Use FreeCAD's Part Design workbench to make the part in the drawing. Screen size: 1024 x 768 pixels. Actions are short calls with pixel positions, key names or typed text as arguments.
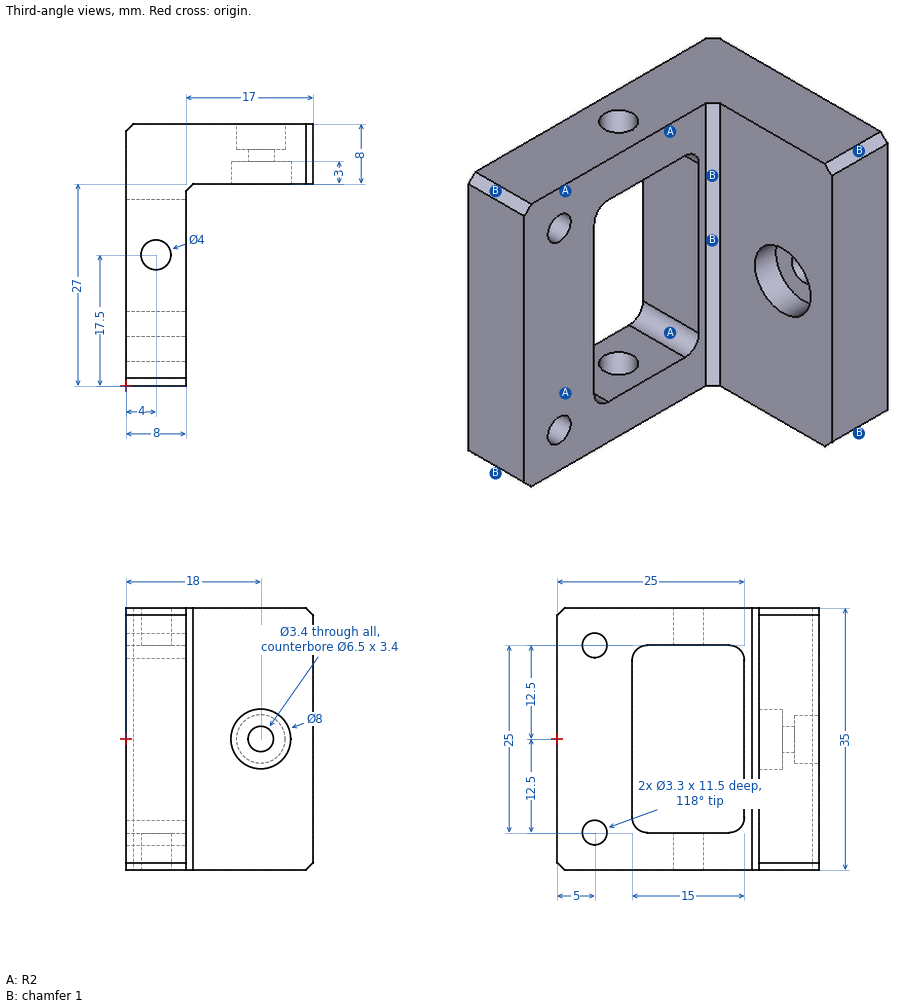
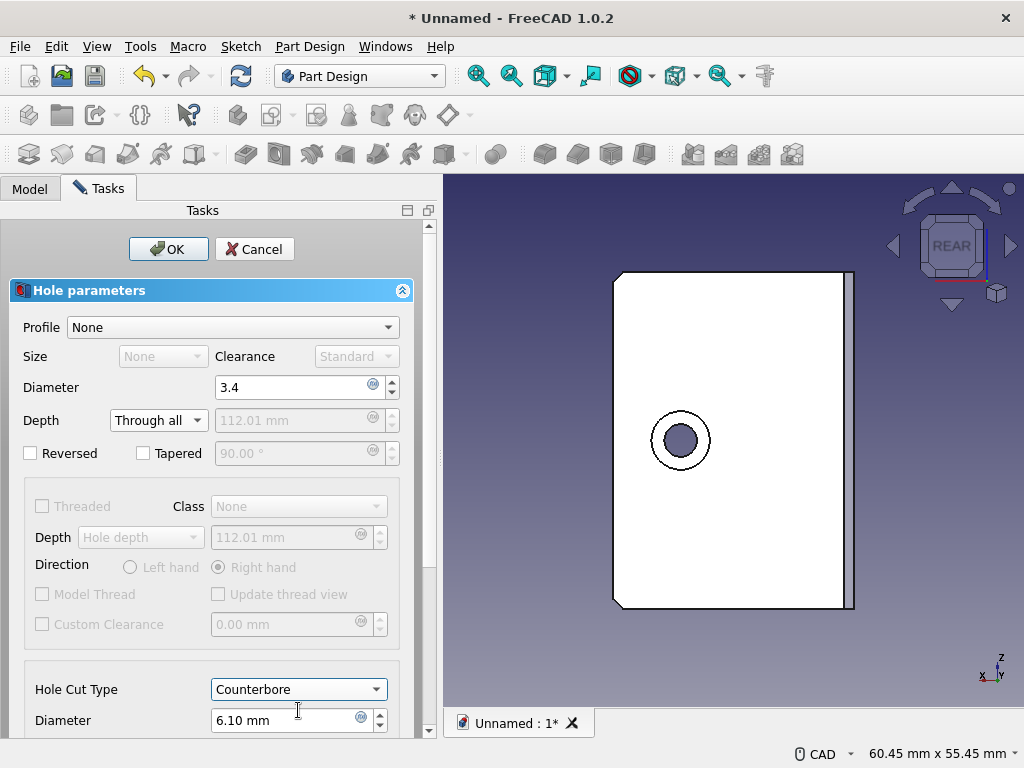
triple_click(292, 720)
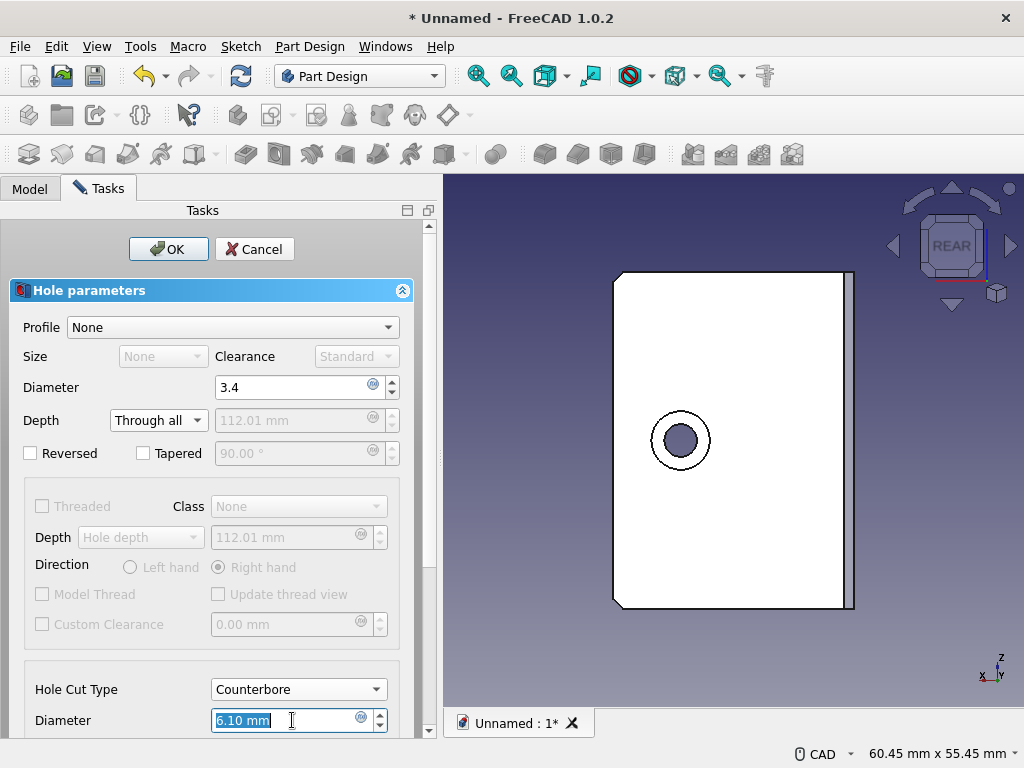
text(6.5)
key(Tab)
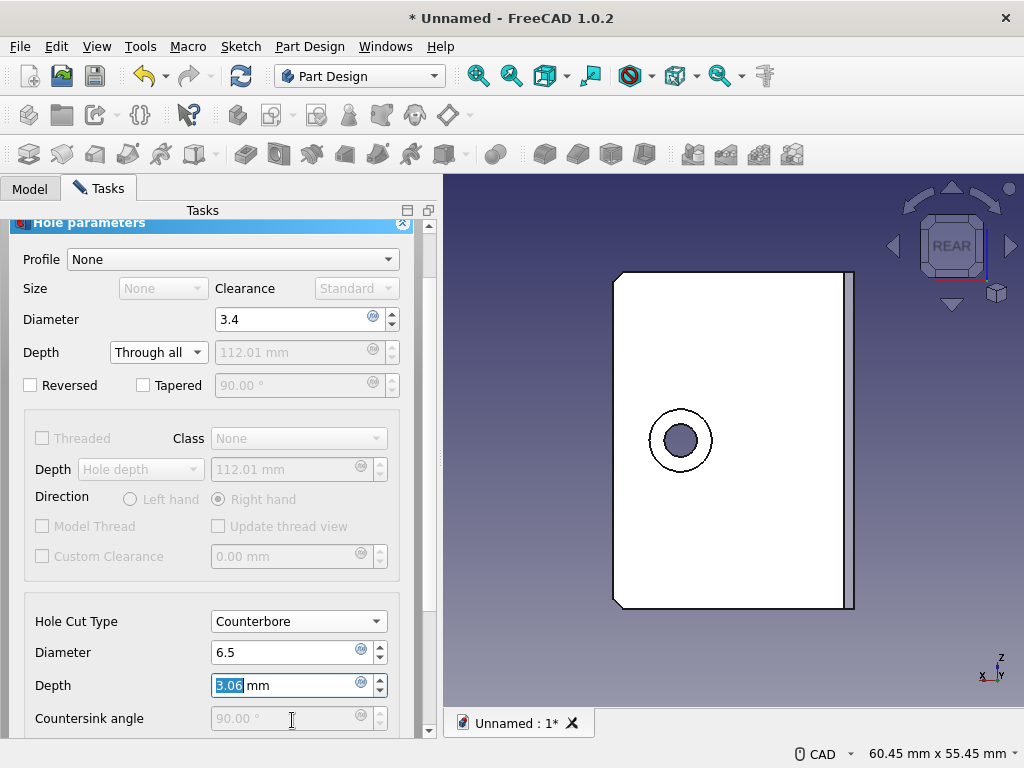
text(3.4)
key(Tab)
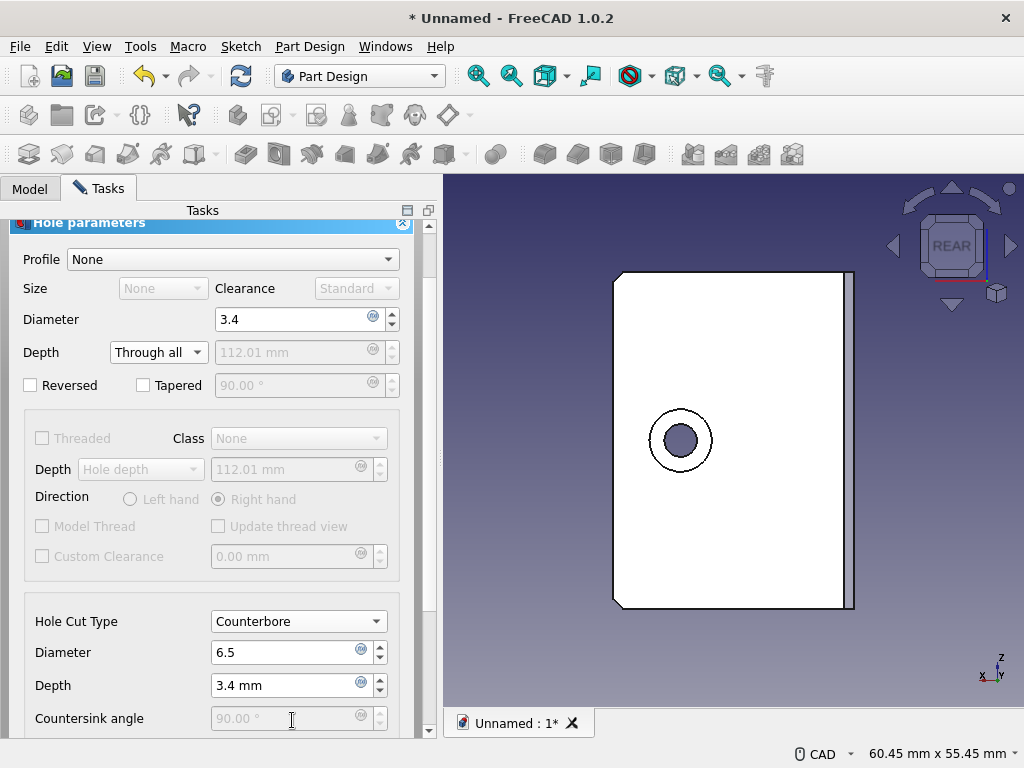
scroll(429, 479, up, 2)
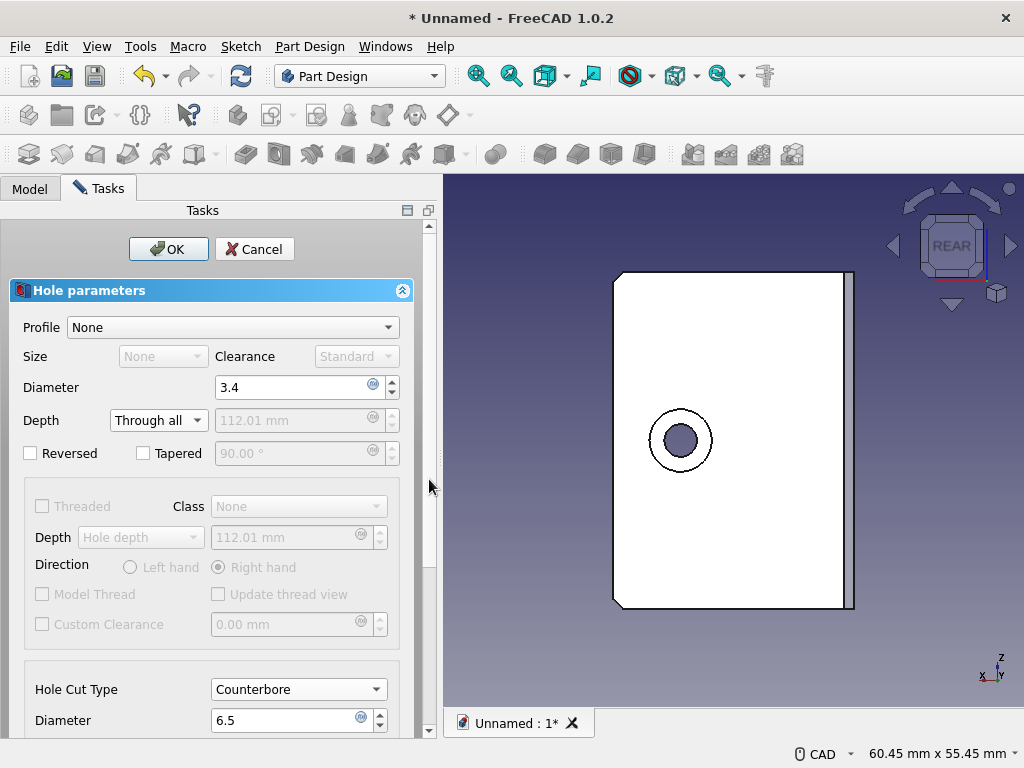
click(169, 249)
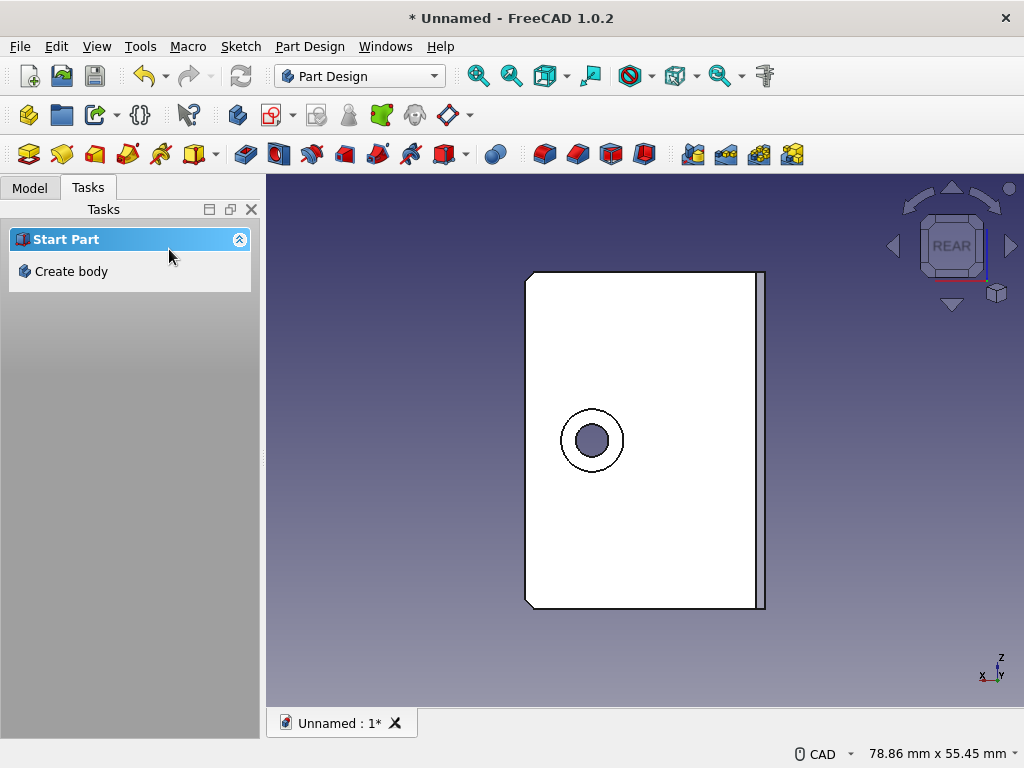
key(0)